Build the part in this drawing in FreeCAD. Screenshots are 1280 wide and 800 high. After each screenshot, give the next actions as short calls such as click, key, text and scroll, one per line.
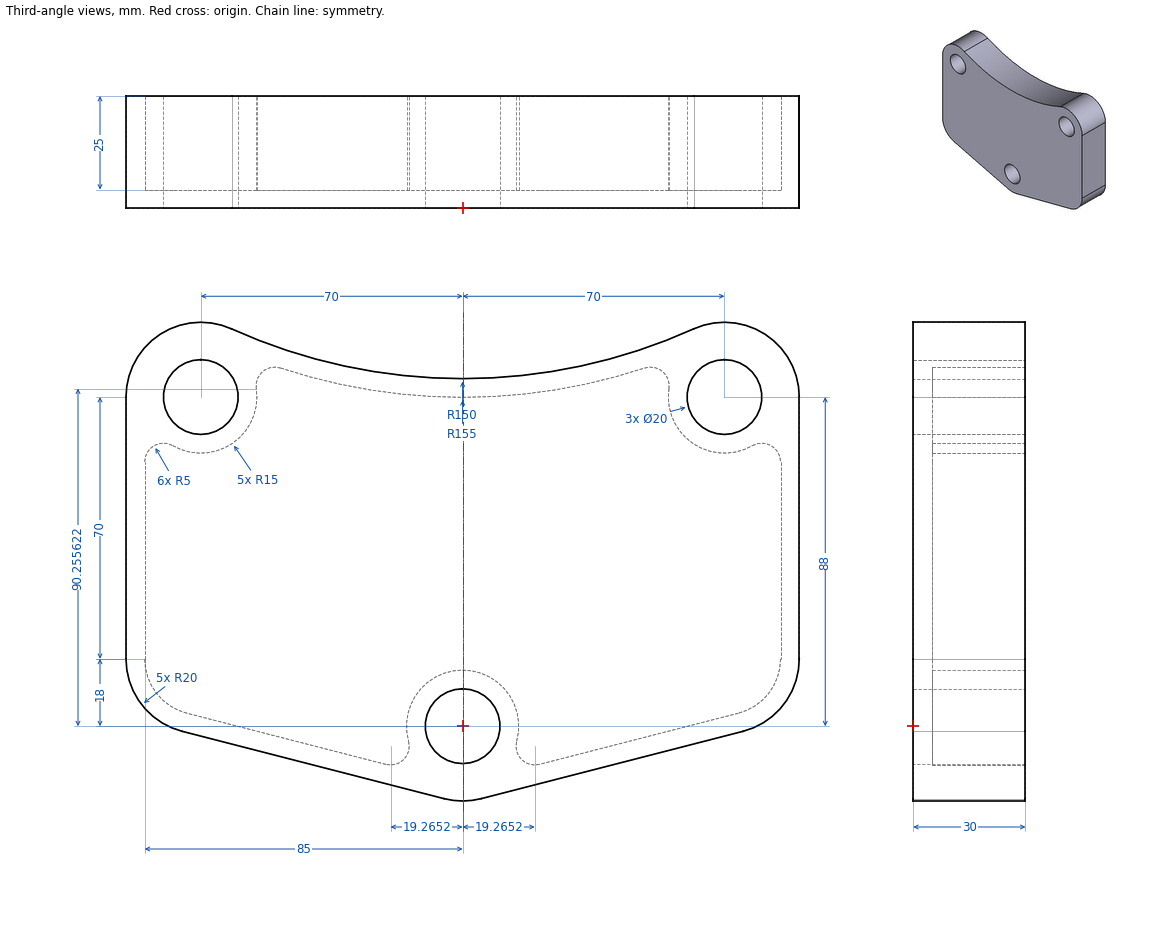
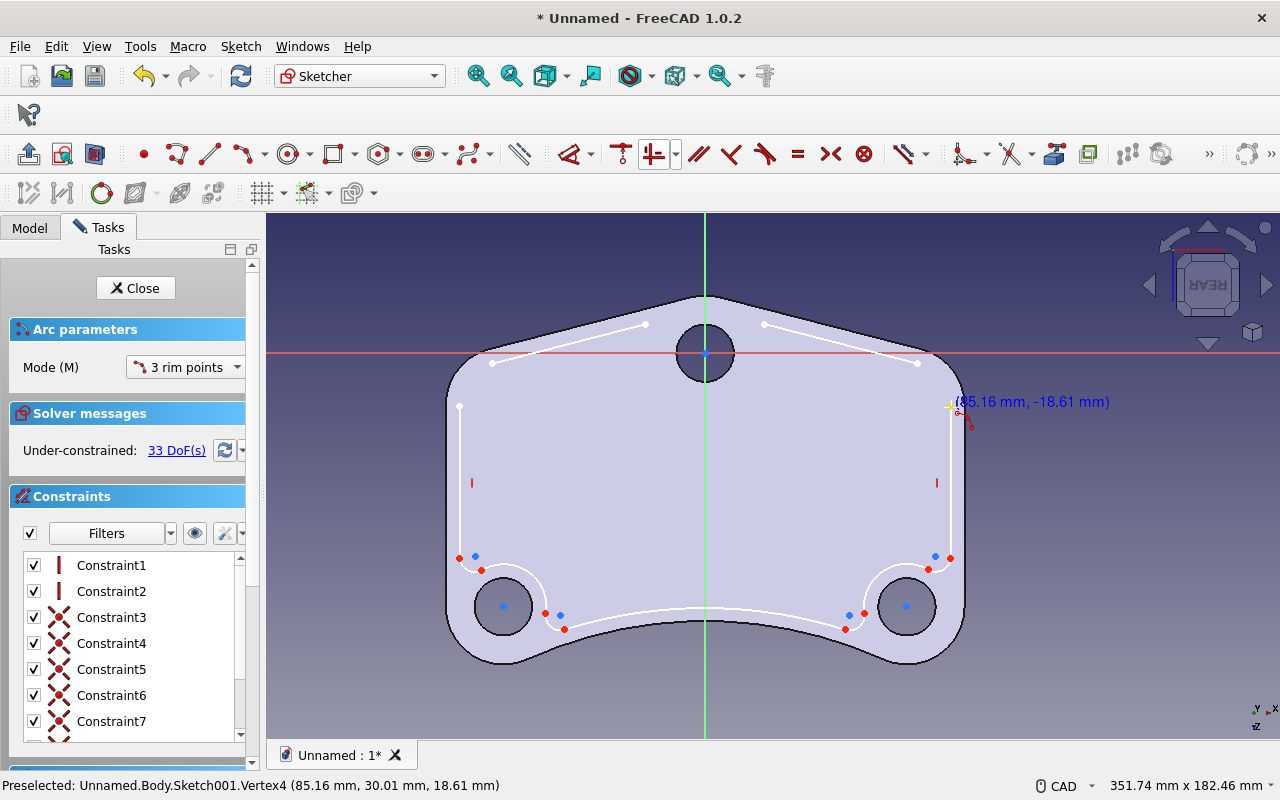
scroll(918, 363, up, 3)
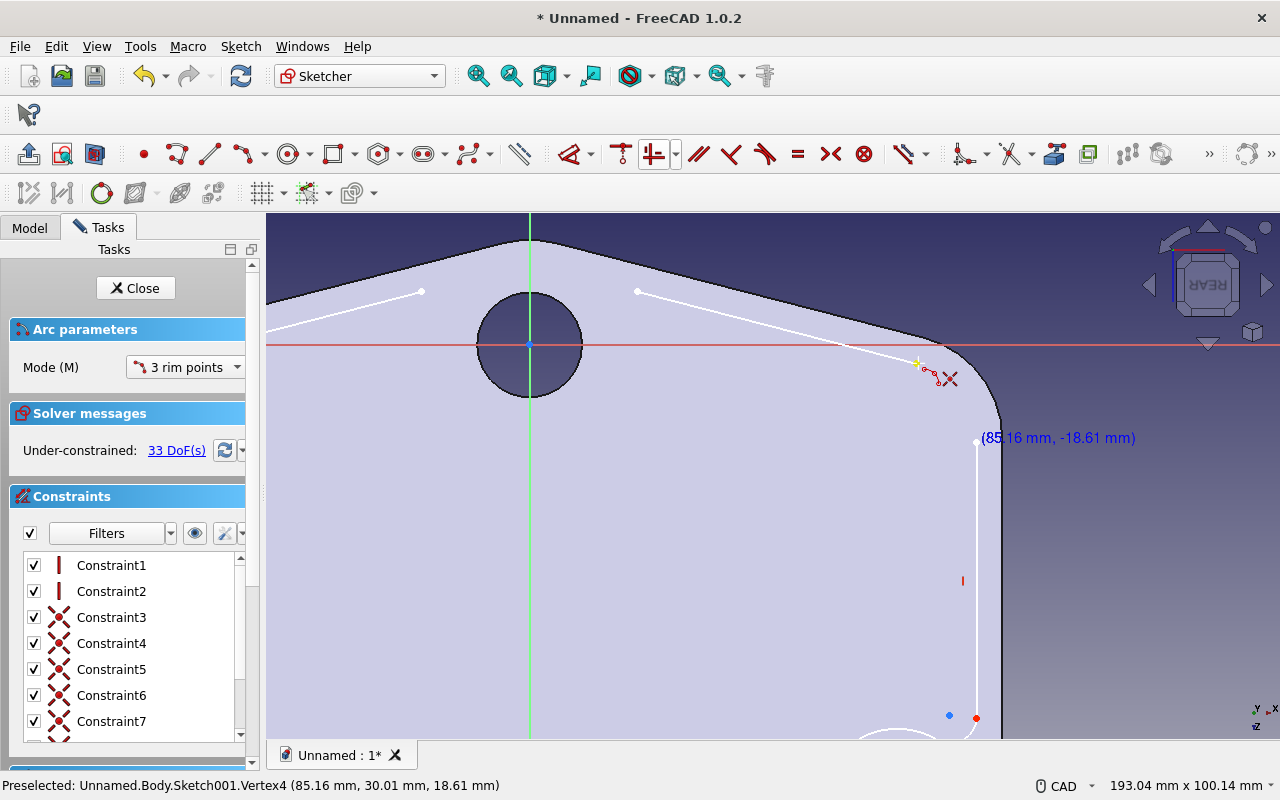
click(917, 364)
click(960, 391)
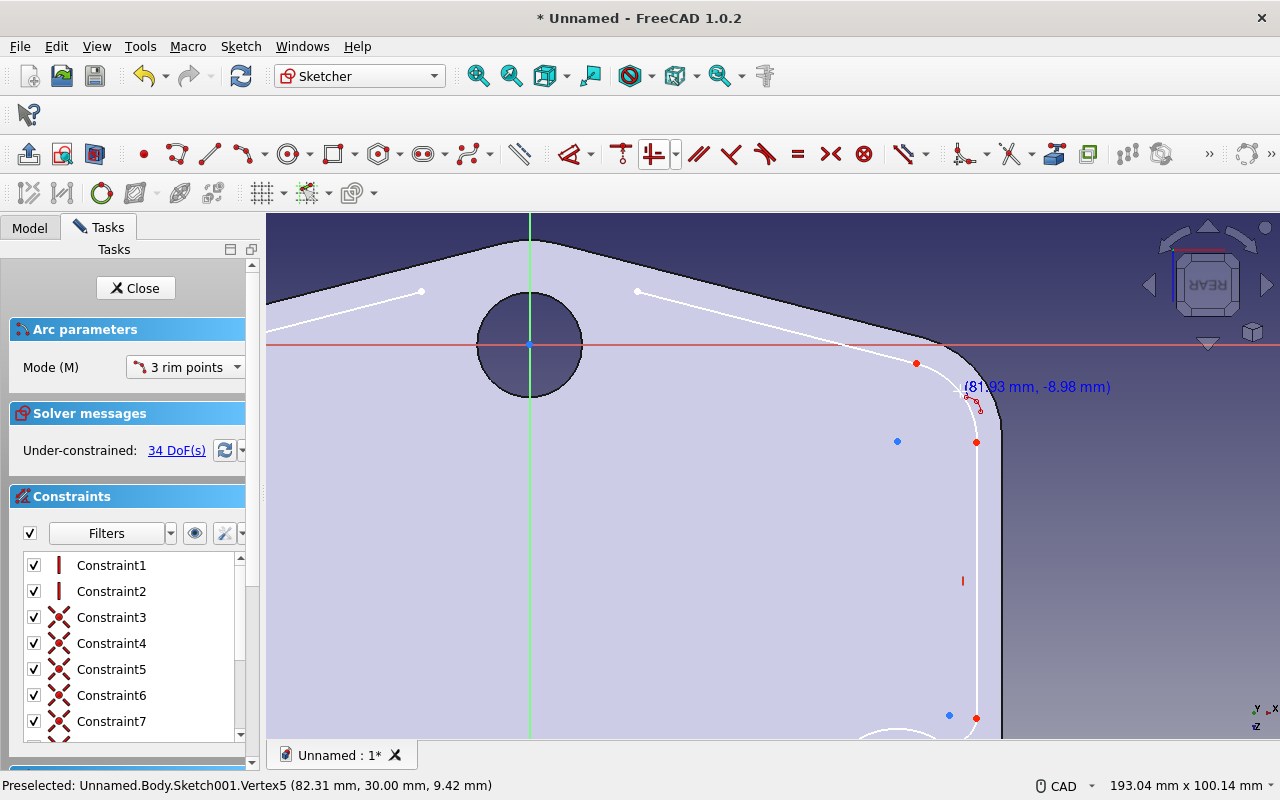
click(638, 292)
click(606, 324)
click(612, 298)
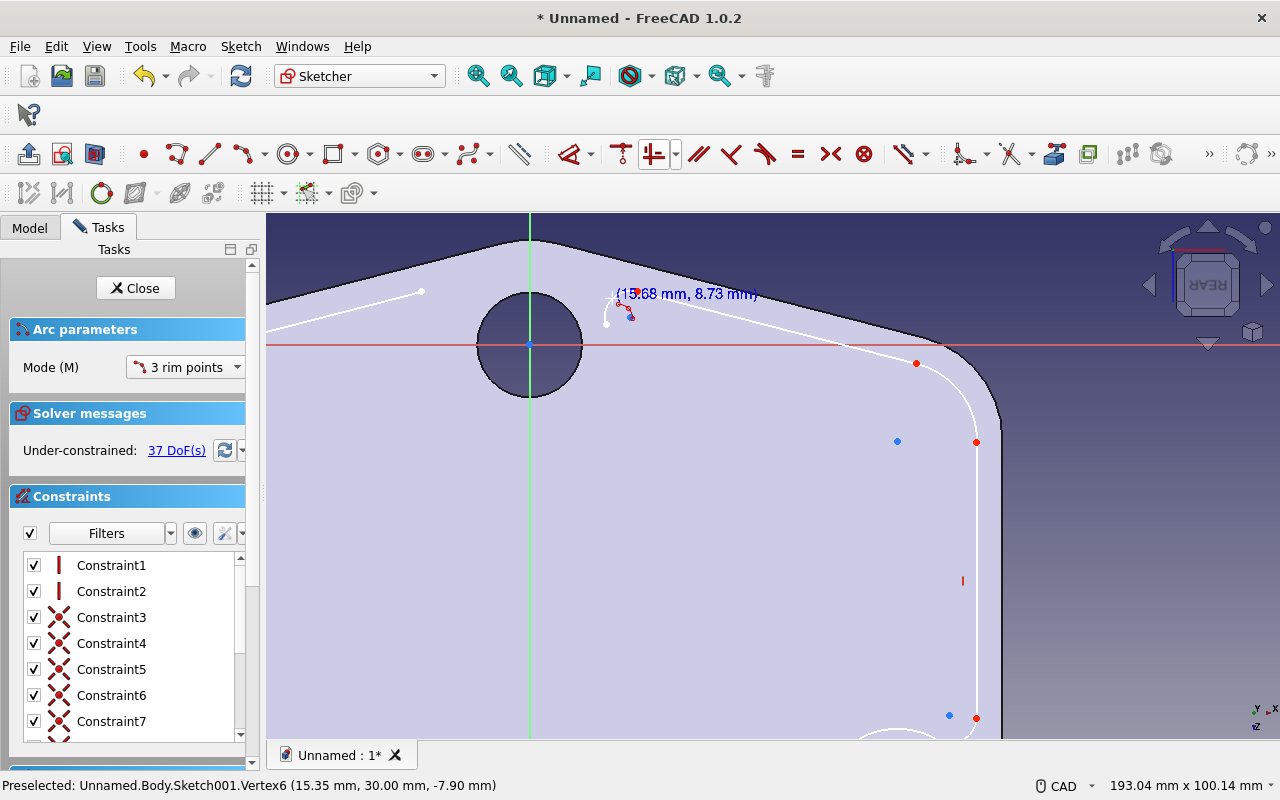
click(606, 325)
click(454, 324)
click(477, 403)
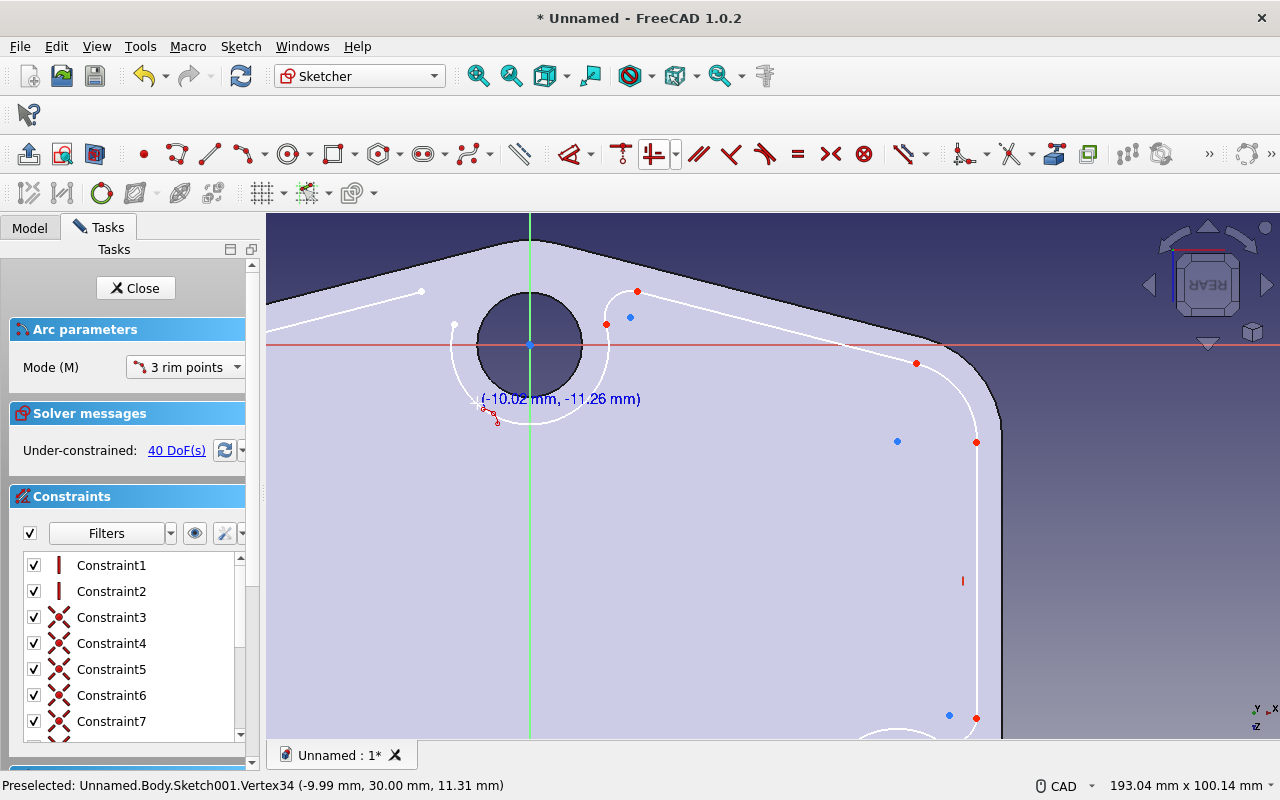
click(454, 325)
click(422, 292)
click(447, 298)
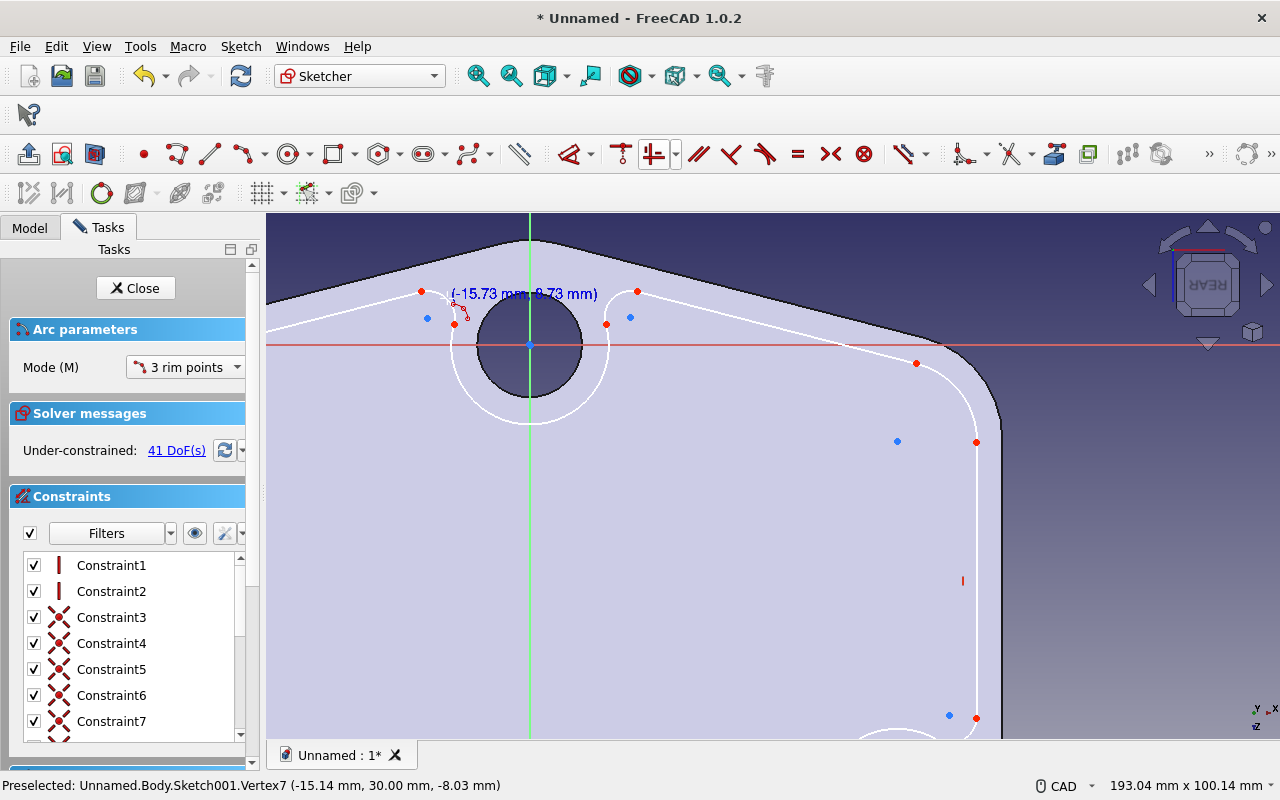
scroll(917, 362, down, 3)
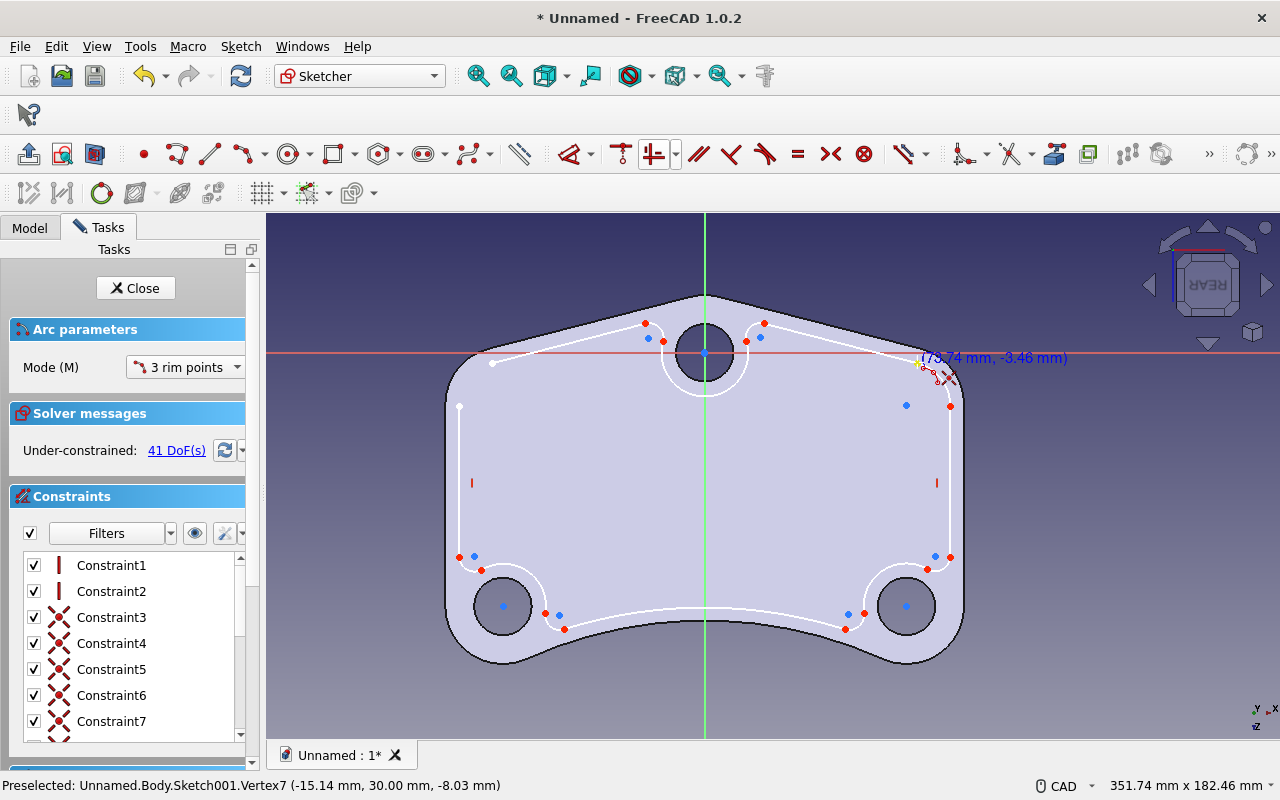
scroll(492, 363, up, 3)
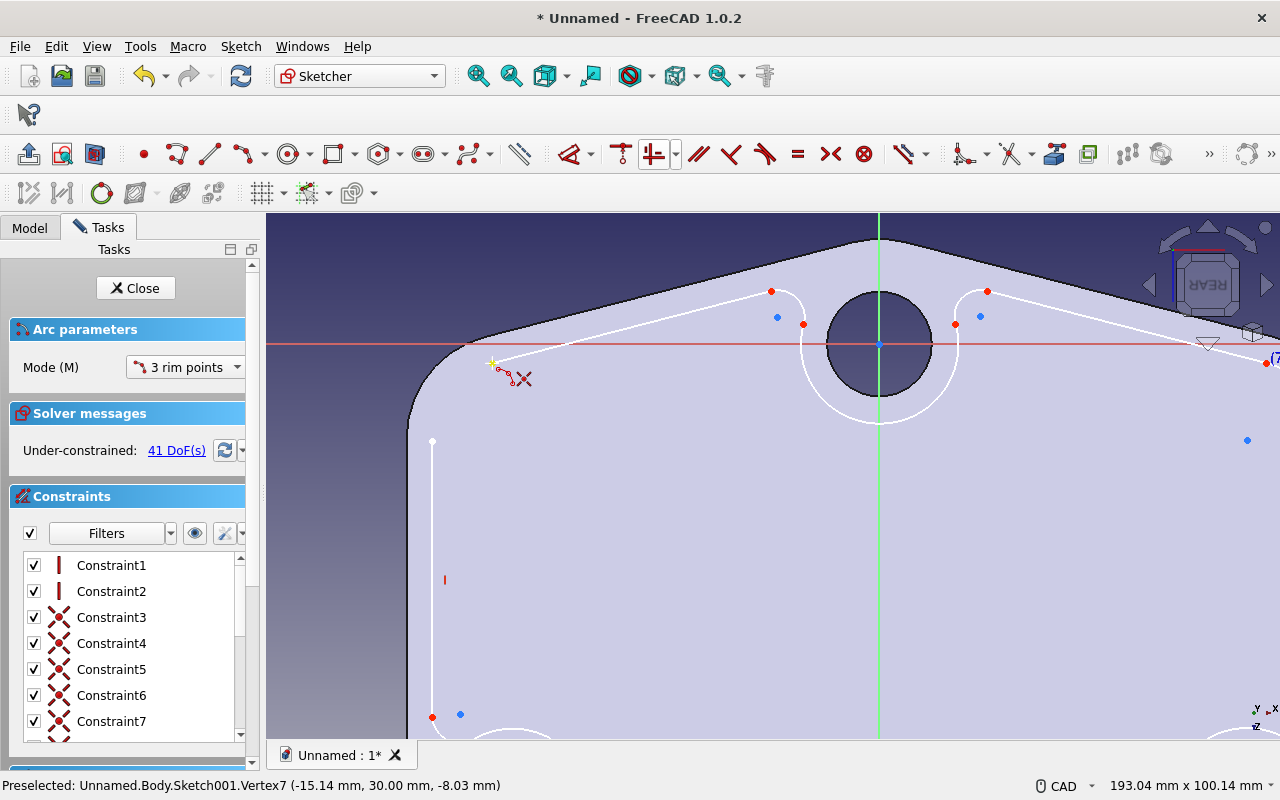
click(493, 363)
click(432, 442)
click(449, 390)
key(Escape)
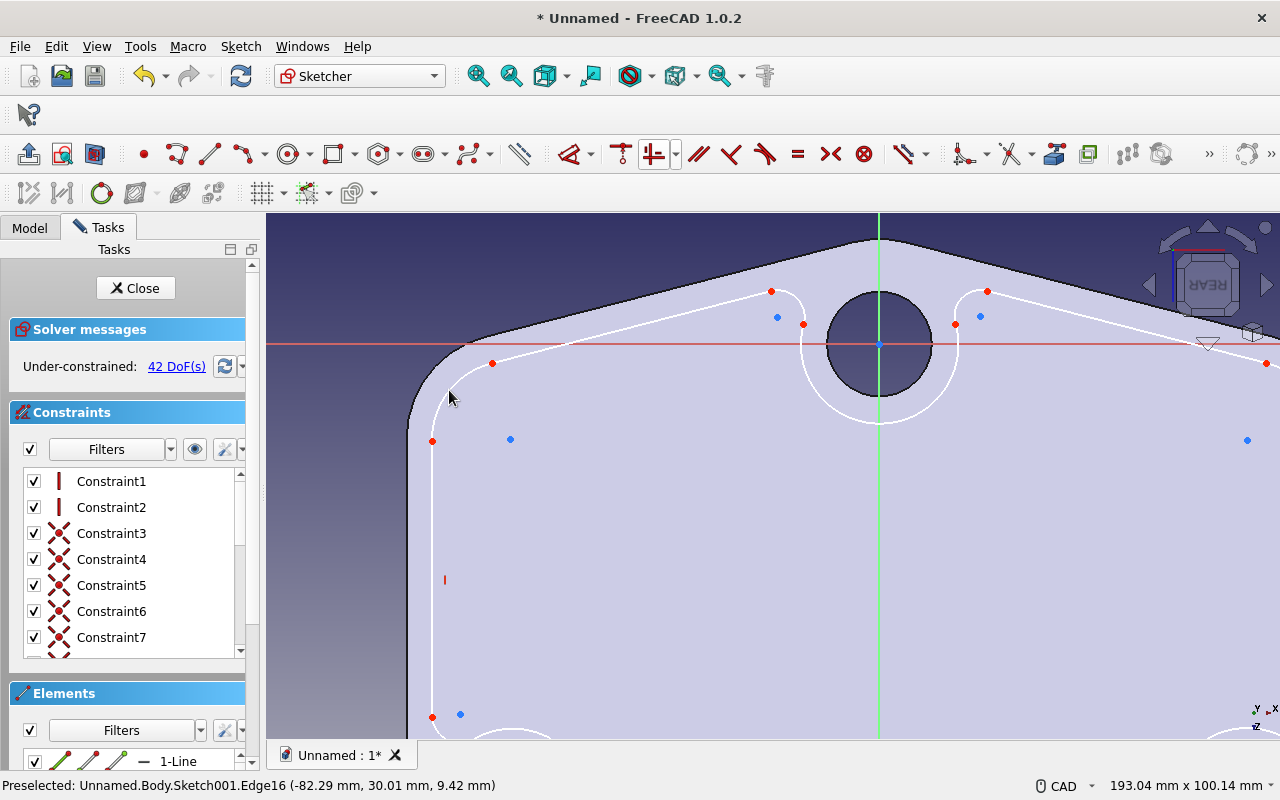
click(432, 525)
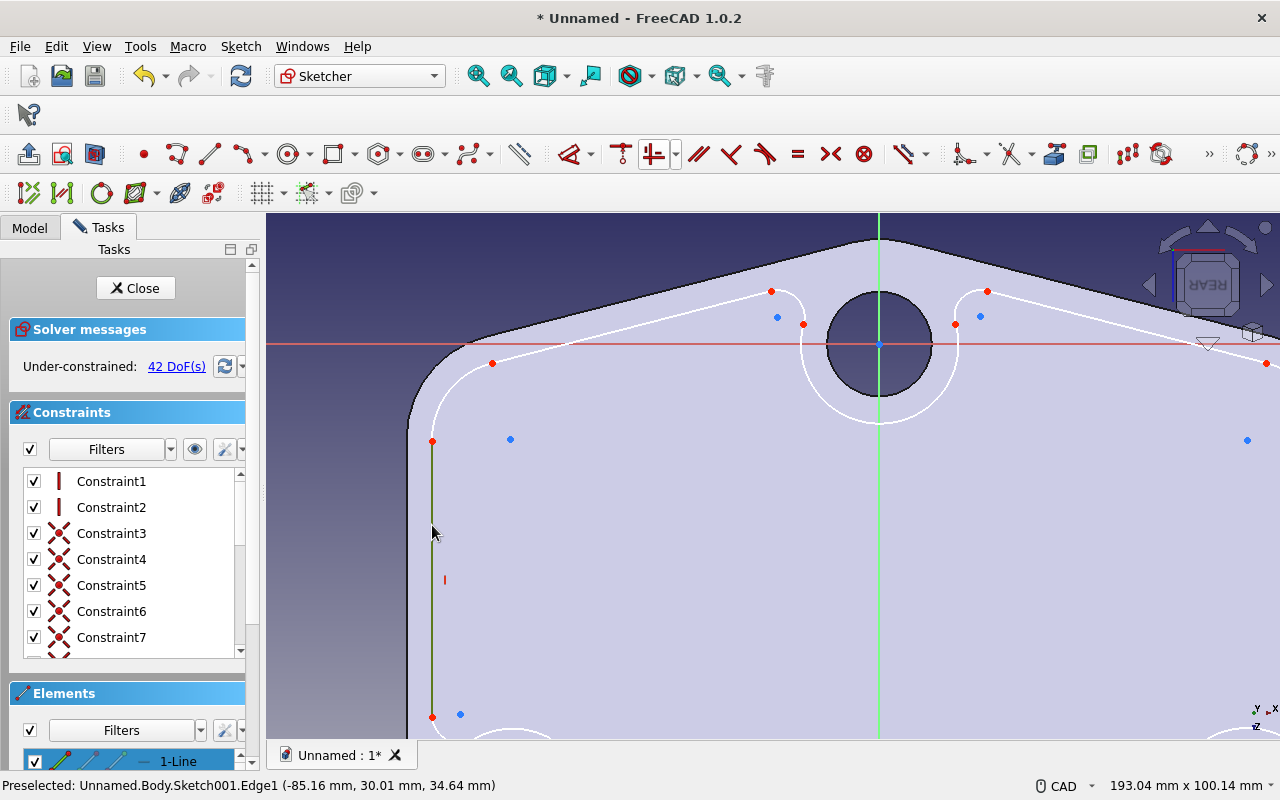
scroll(492, 363, down, 3)